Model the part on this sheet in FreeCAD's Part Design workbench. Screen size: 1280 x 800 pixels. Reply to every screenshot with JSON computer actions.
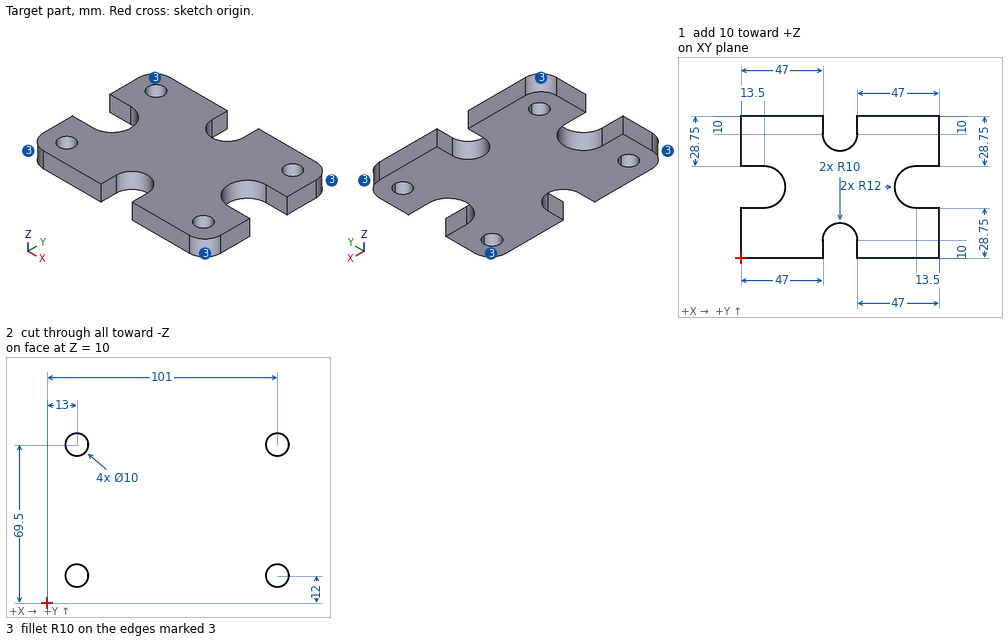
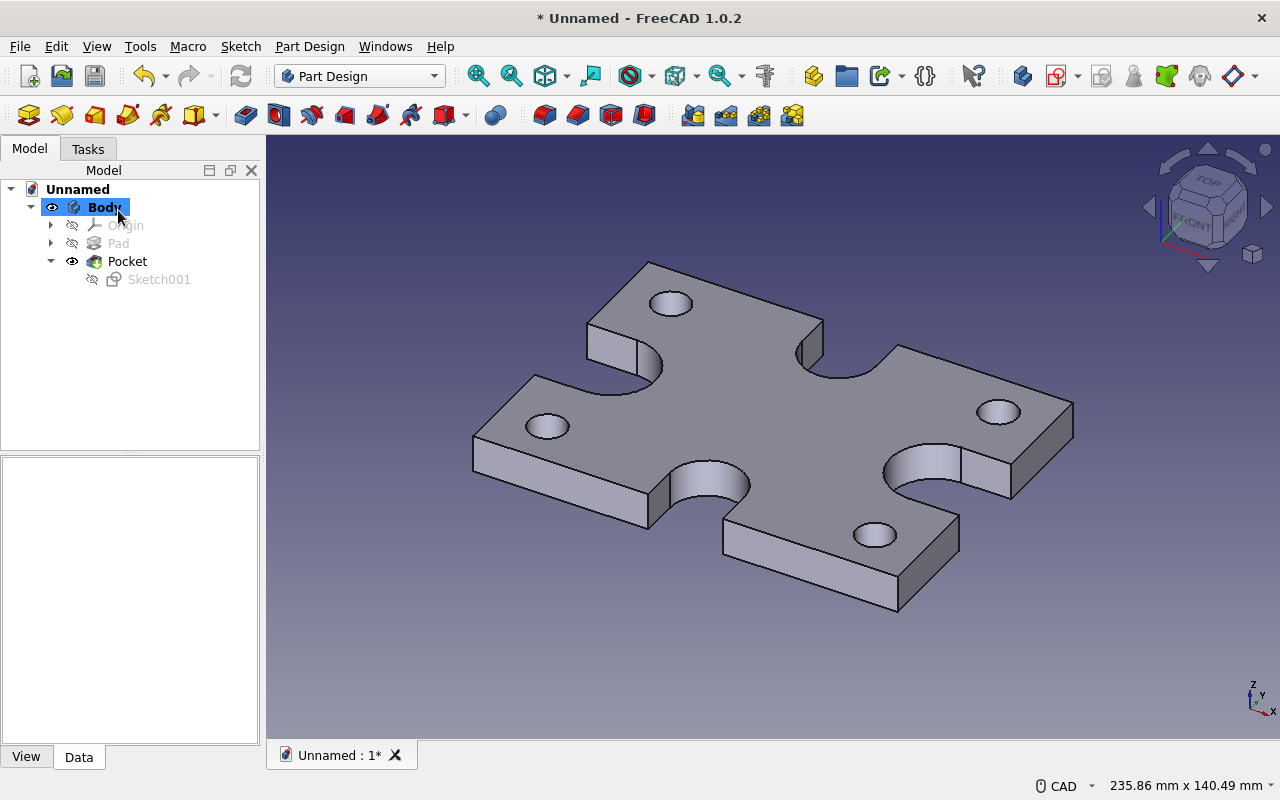
{"action": "left_click", "coordinate": [898, 593]}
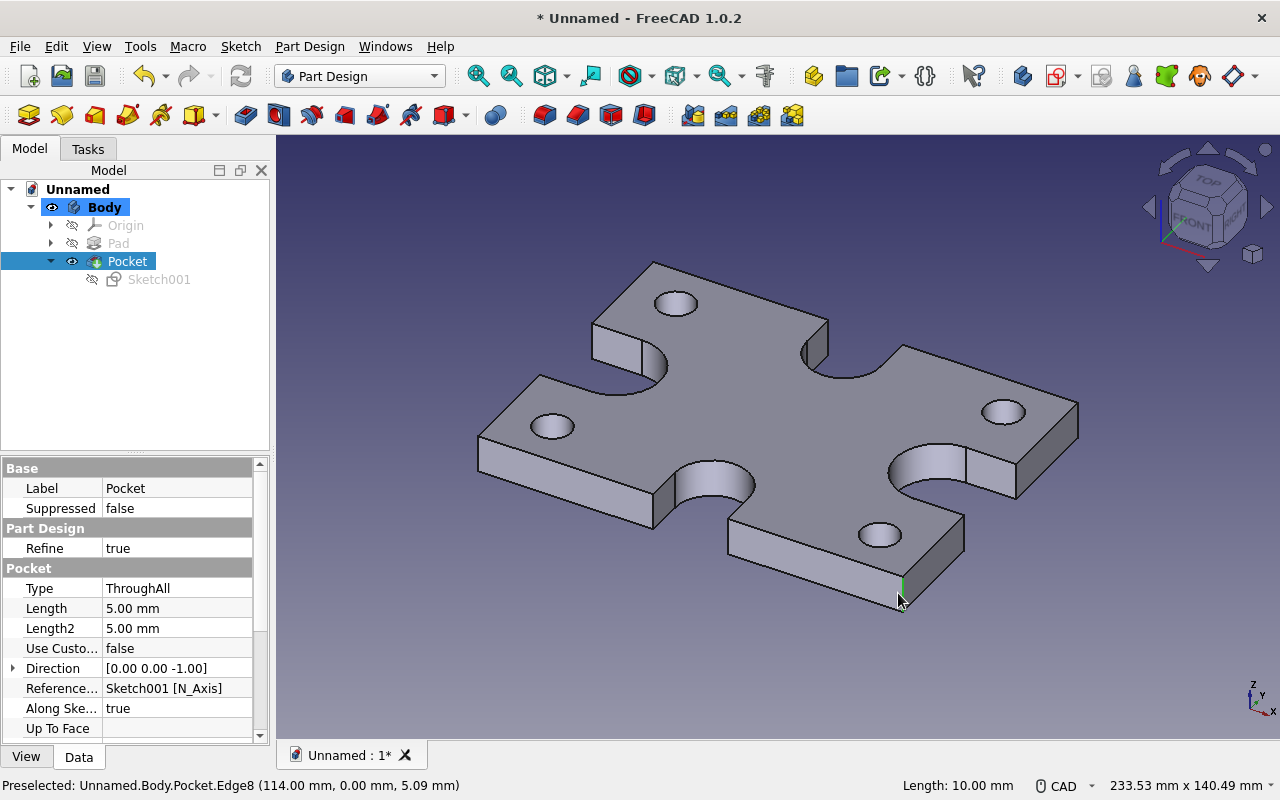
{"action": "key", "text": "0"}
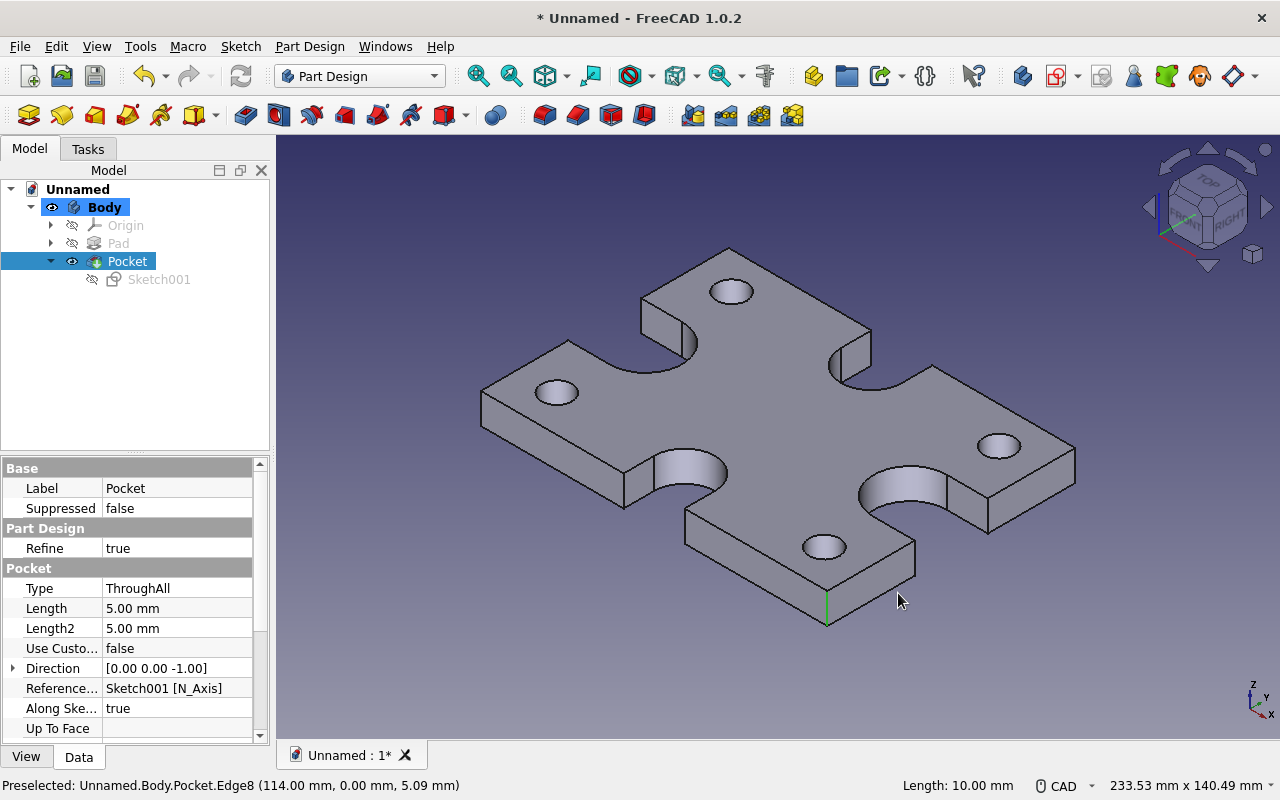
{"action": "key", "text": "2"}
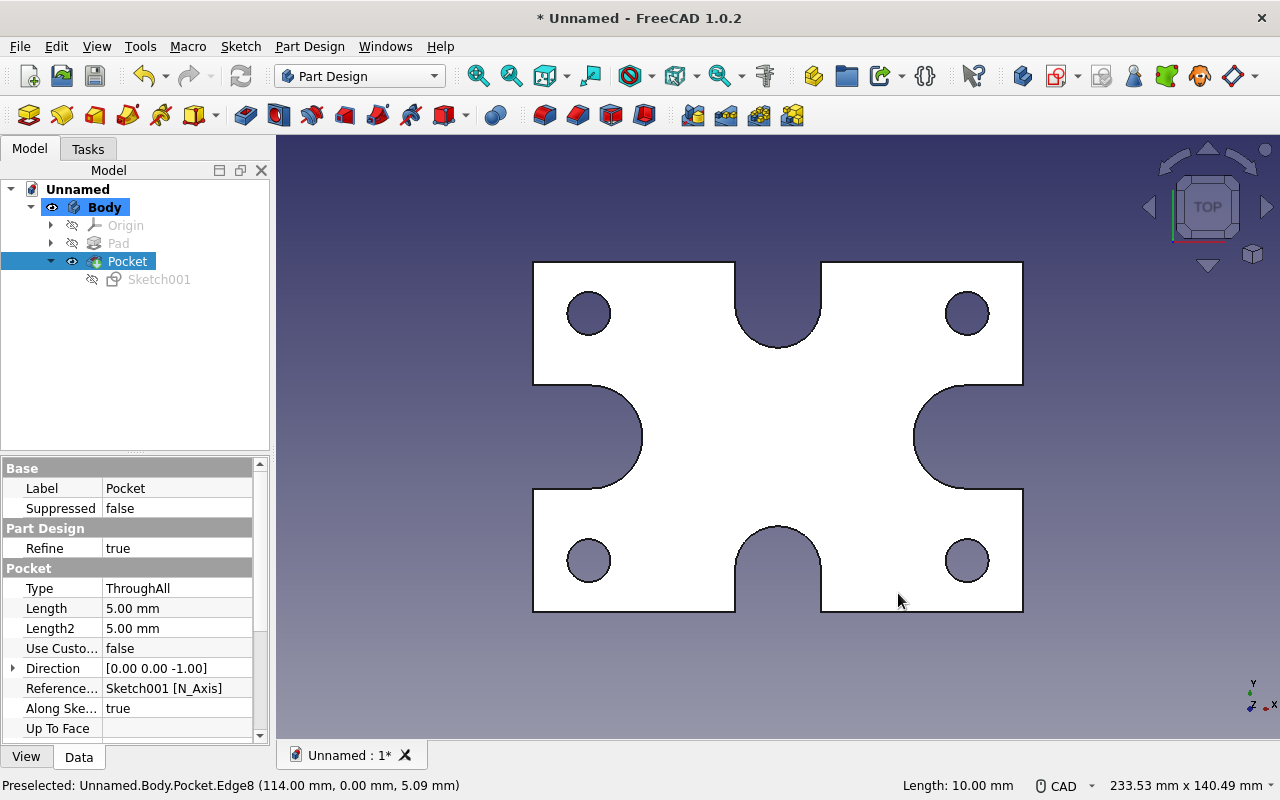
{"action": "key", "text": "1"}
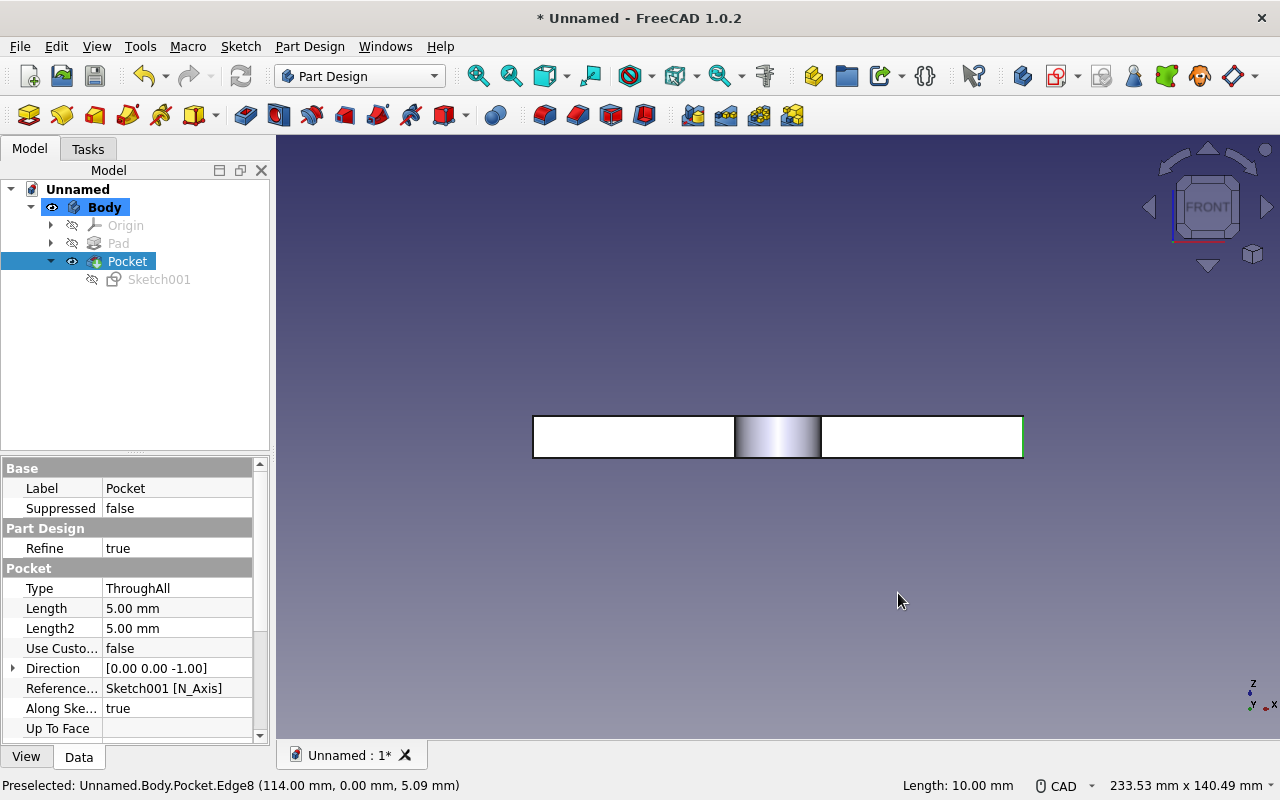
{"action": "left_click", "coordinate": [533, 436], "text": "ctrl"}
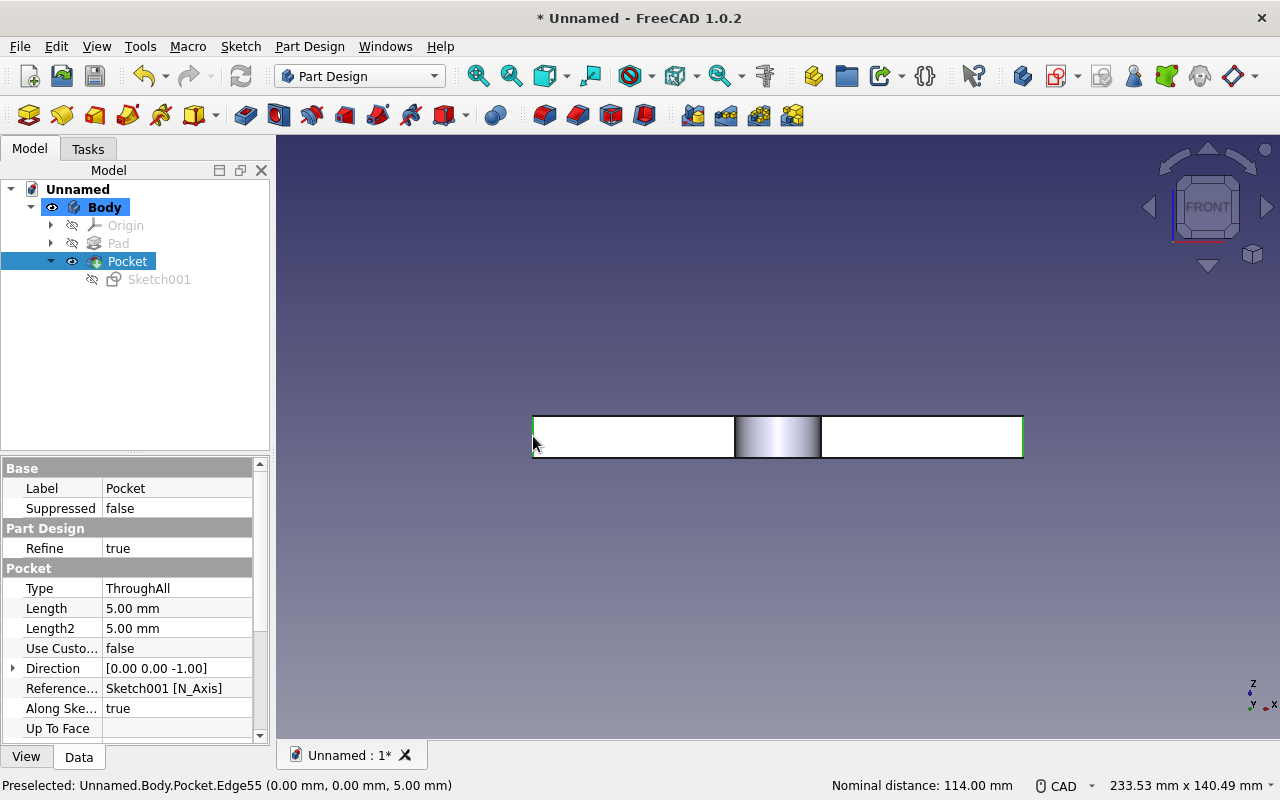
{"action": "key", "text": "3"}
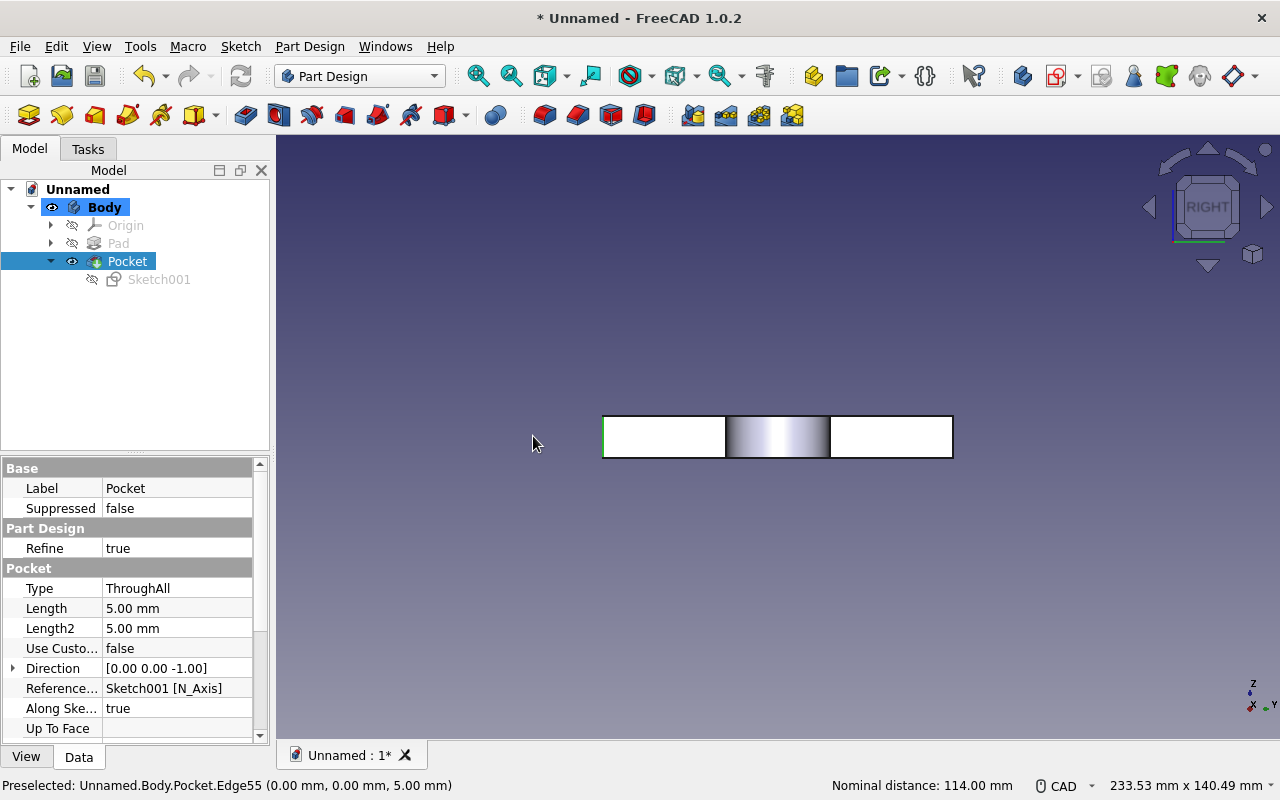
{"action": "left_click", "coordinate": [479, 76]}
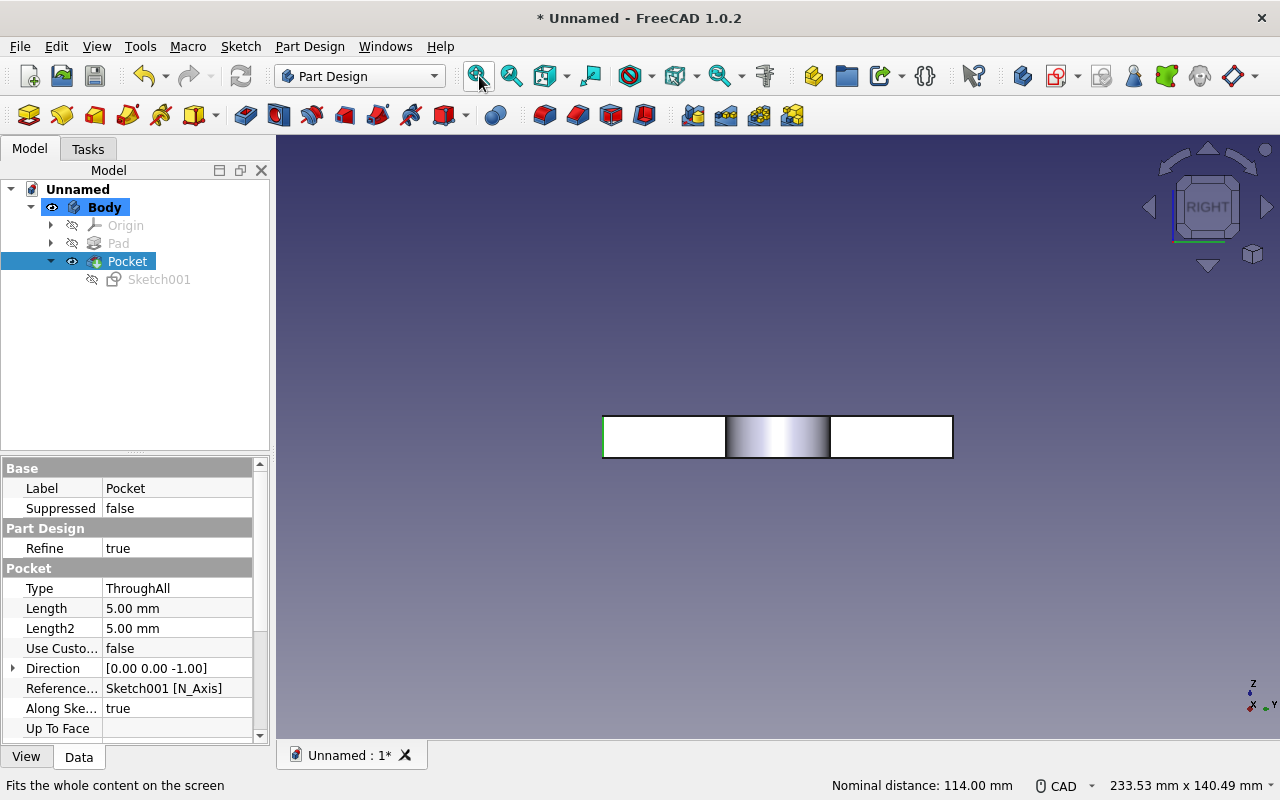
{"action": "left_click", "coordinate": [953, 436], "text": "ctrl"}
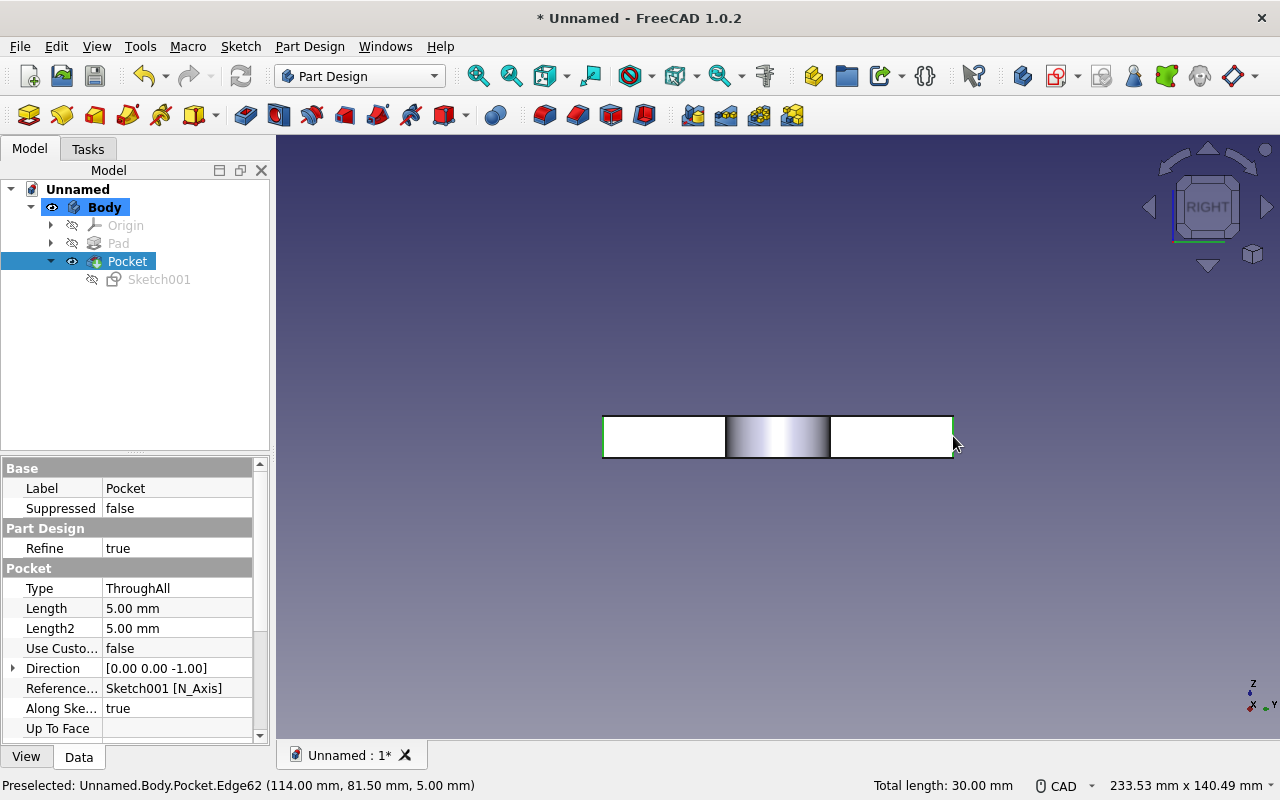
{"action": "key", "text": "5"}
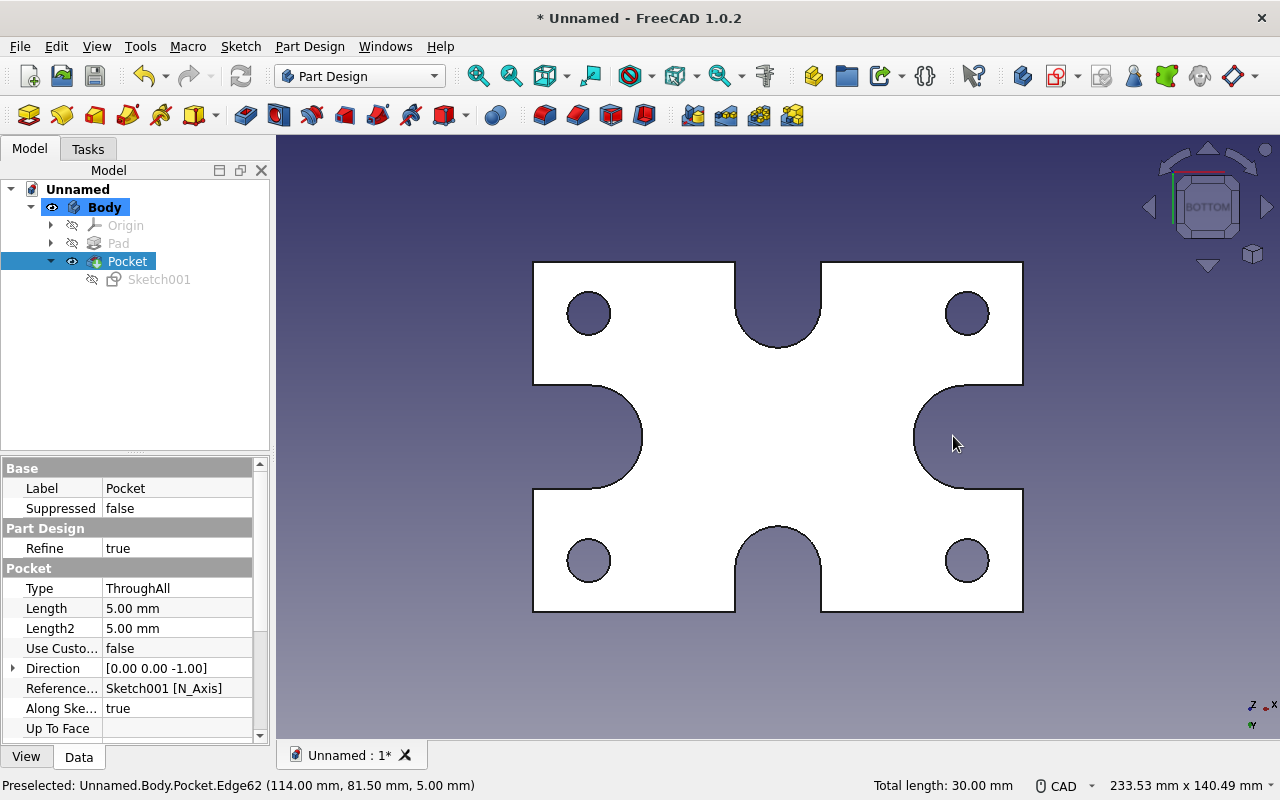
{"action": "key", "text": "4"}